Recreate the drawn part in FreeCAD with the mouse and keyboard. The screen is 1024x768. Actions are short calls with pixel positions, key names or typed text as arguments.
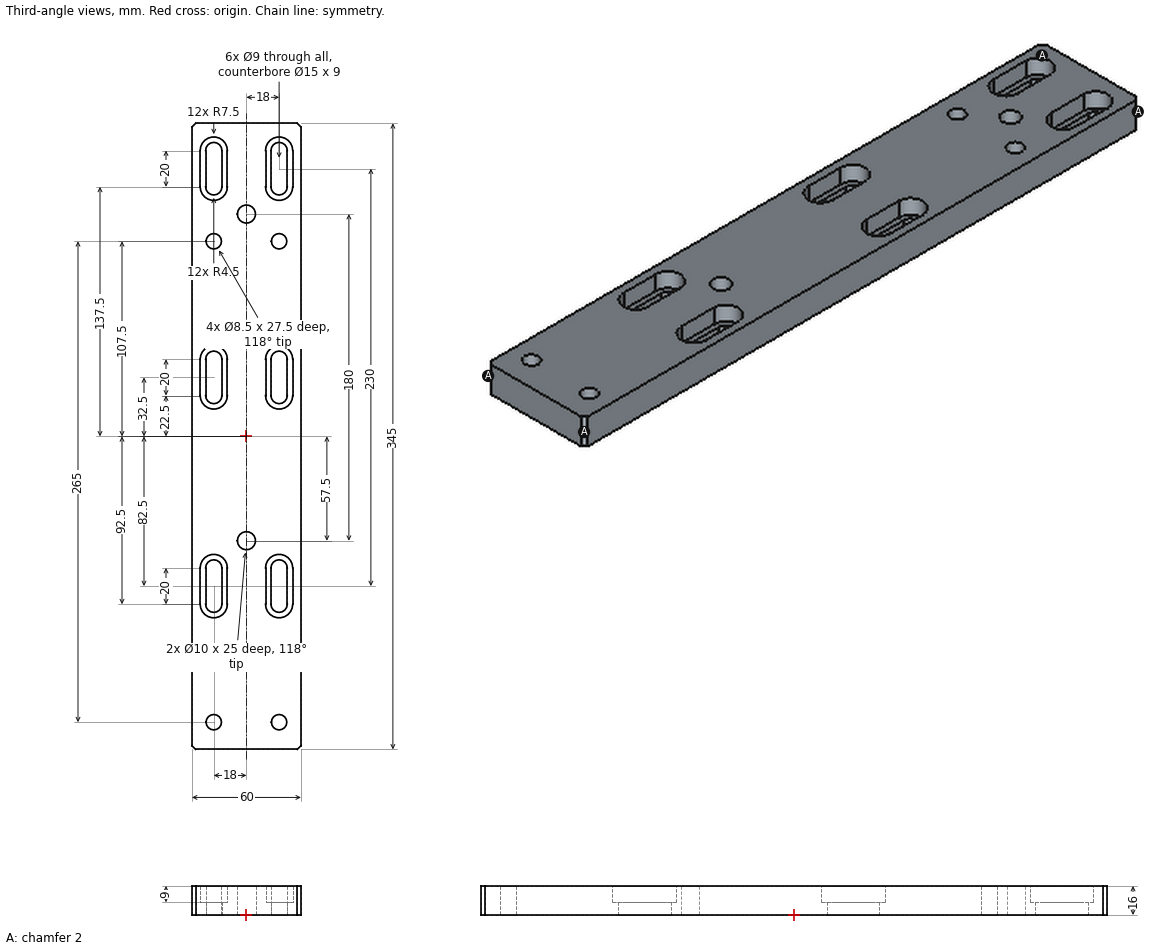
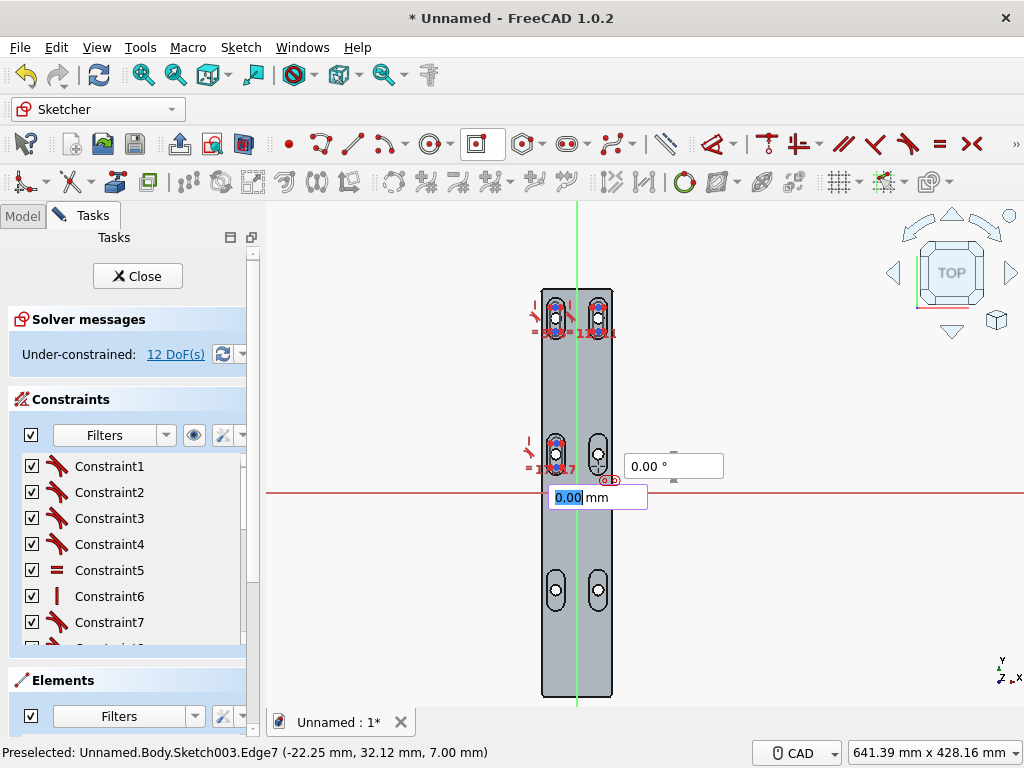
click(598, 443)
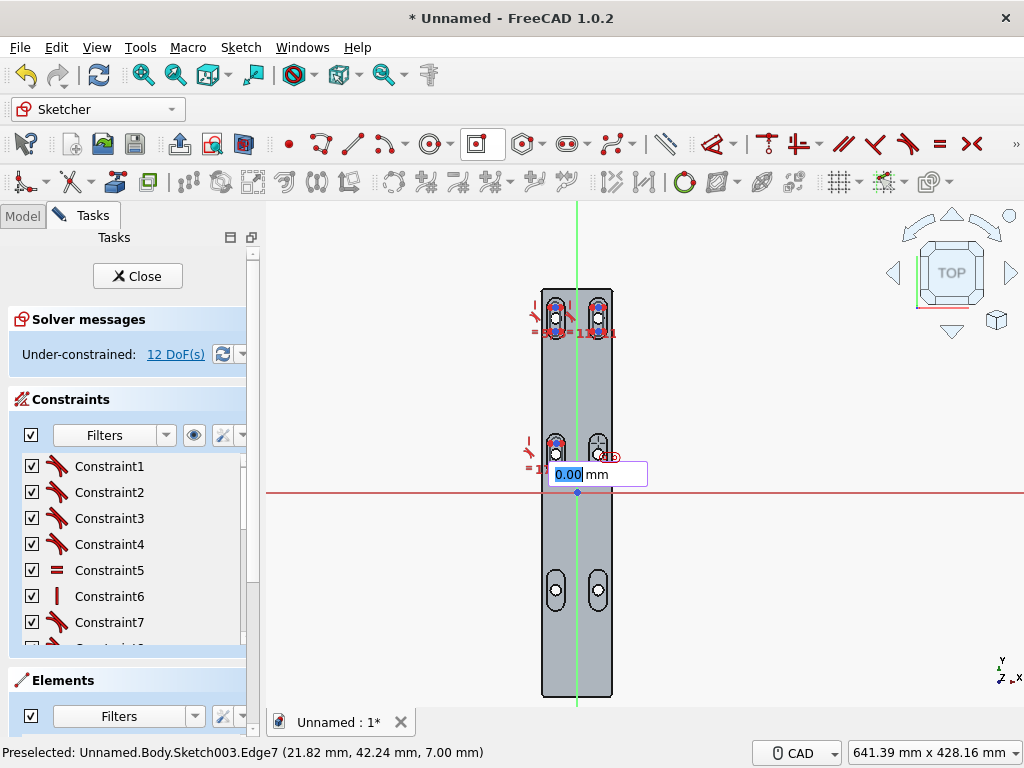
scroll(593, 454, up, 6)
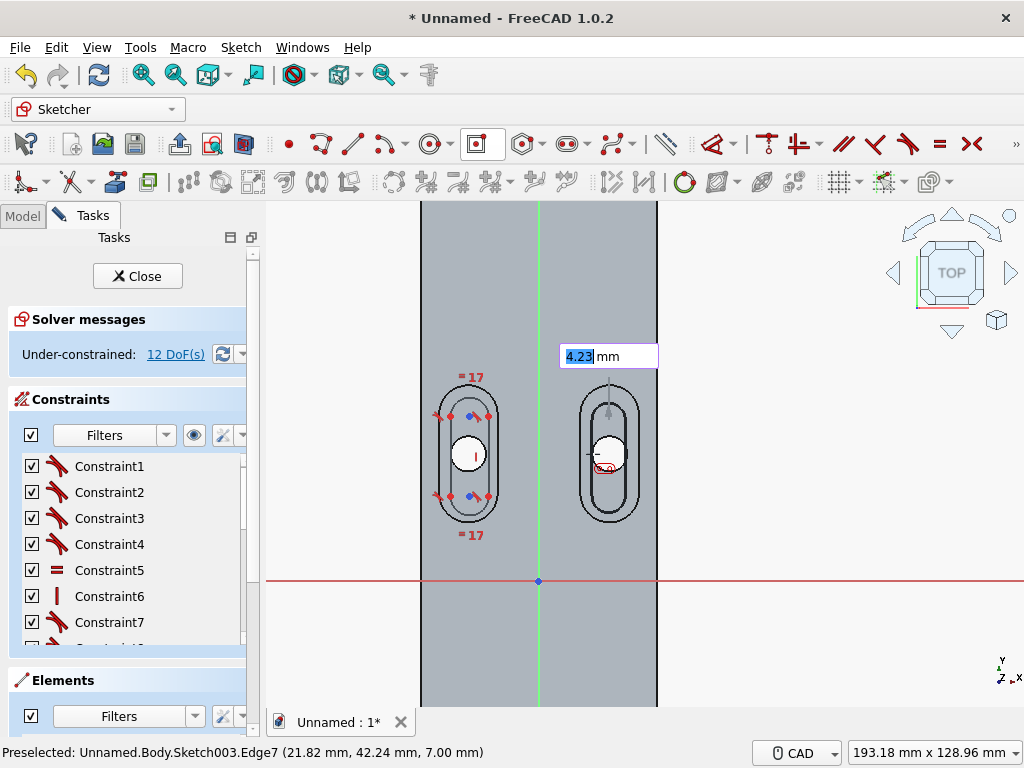
click(592, 454)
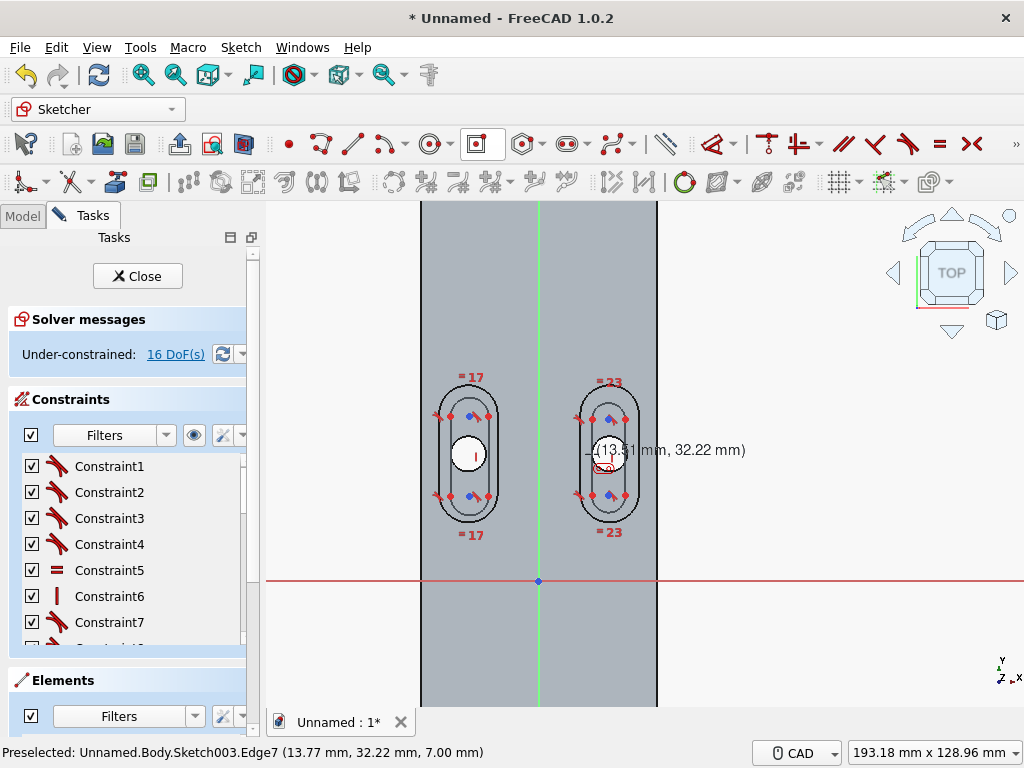
scroll(593, 454, down, 6)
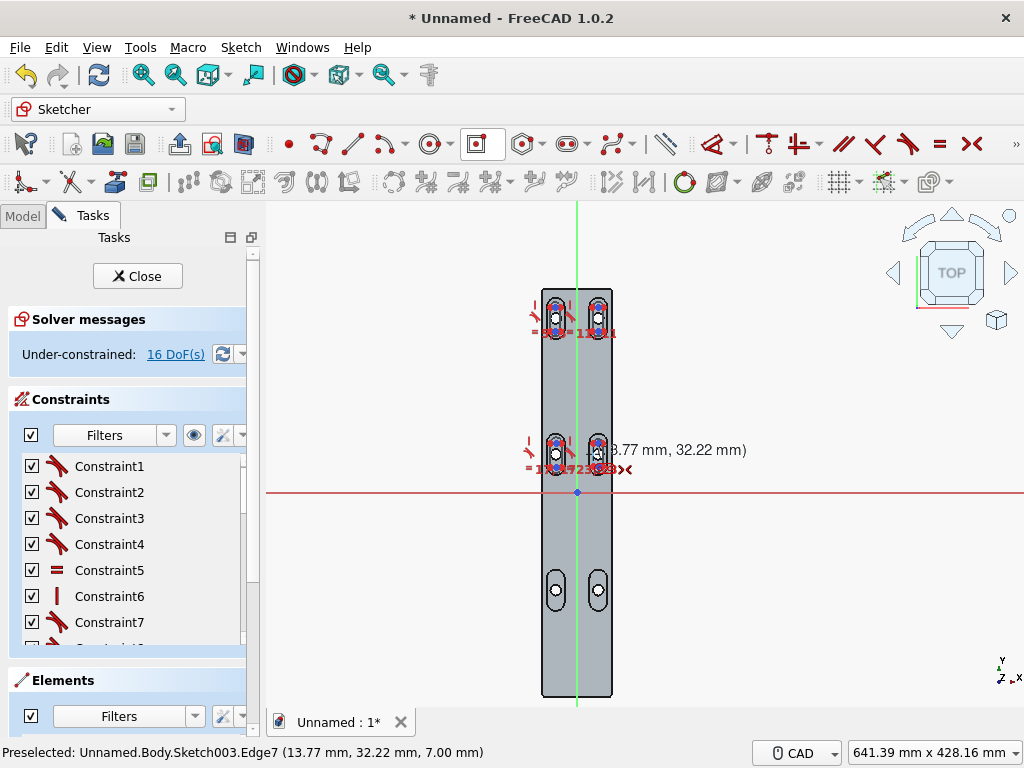
scroll(556, 602, up, 8)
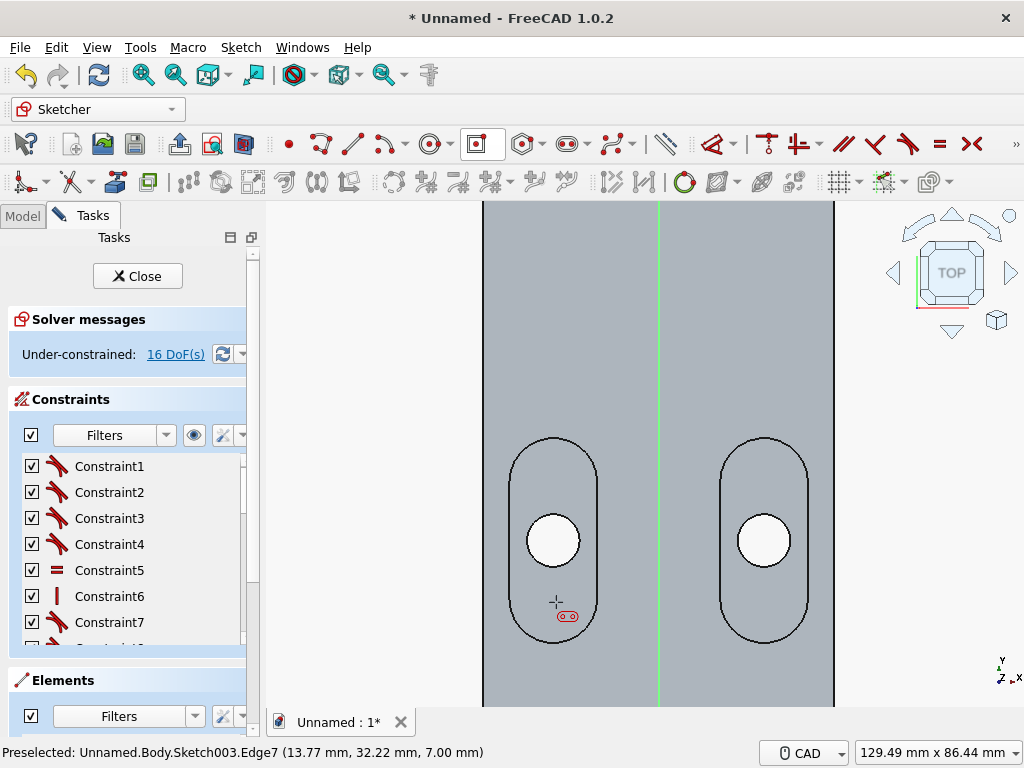
scroll(556, 602, down, 8)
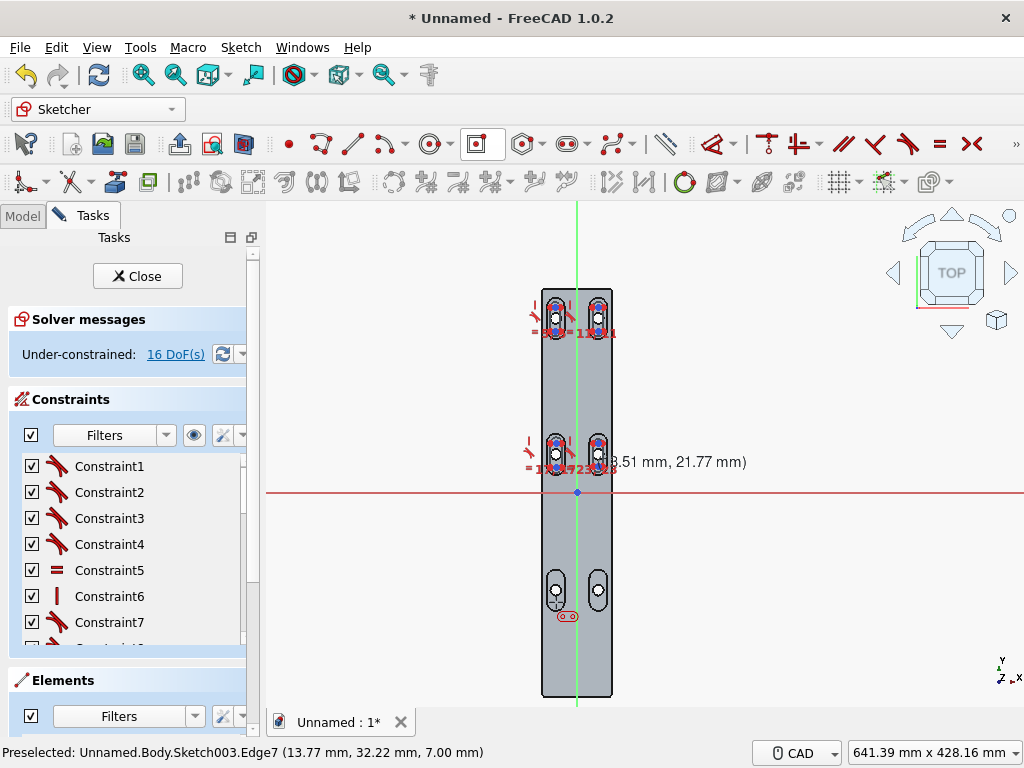
click(556, 602)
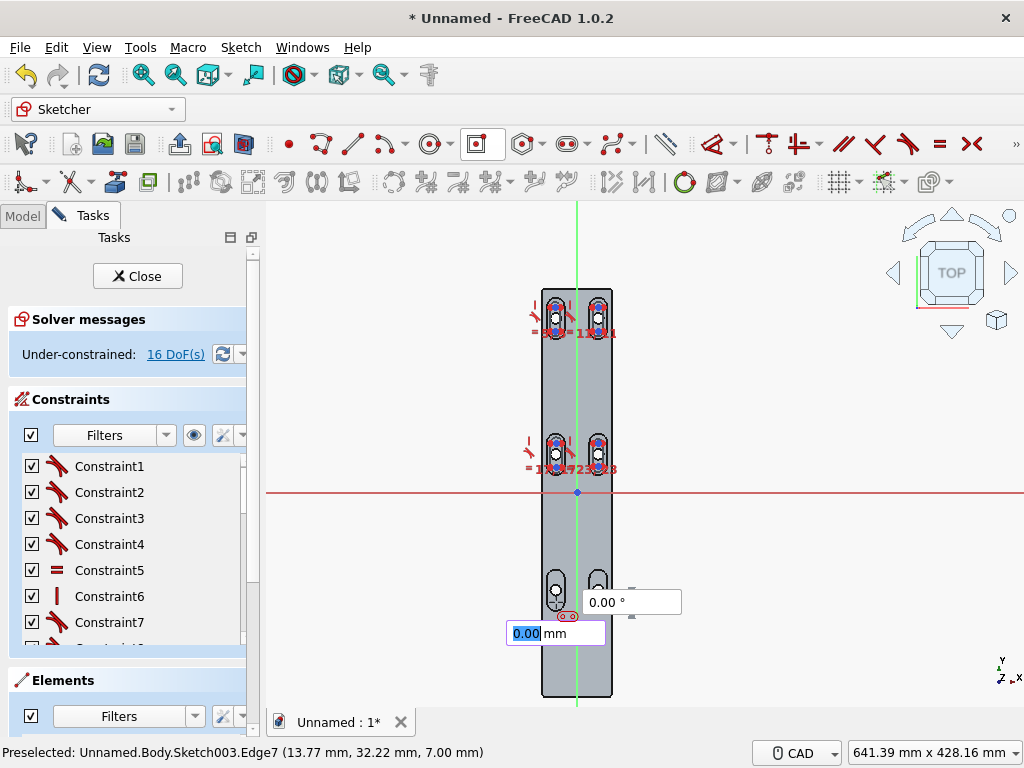
click(556, 578)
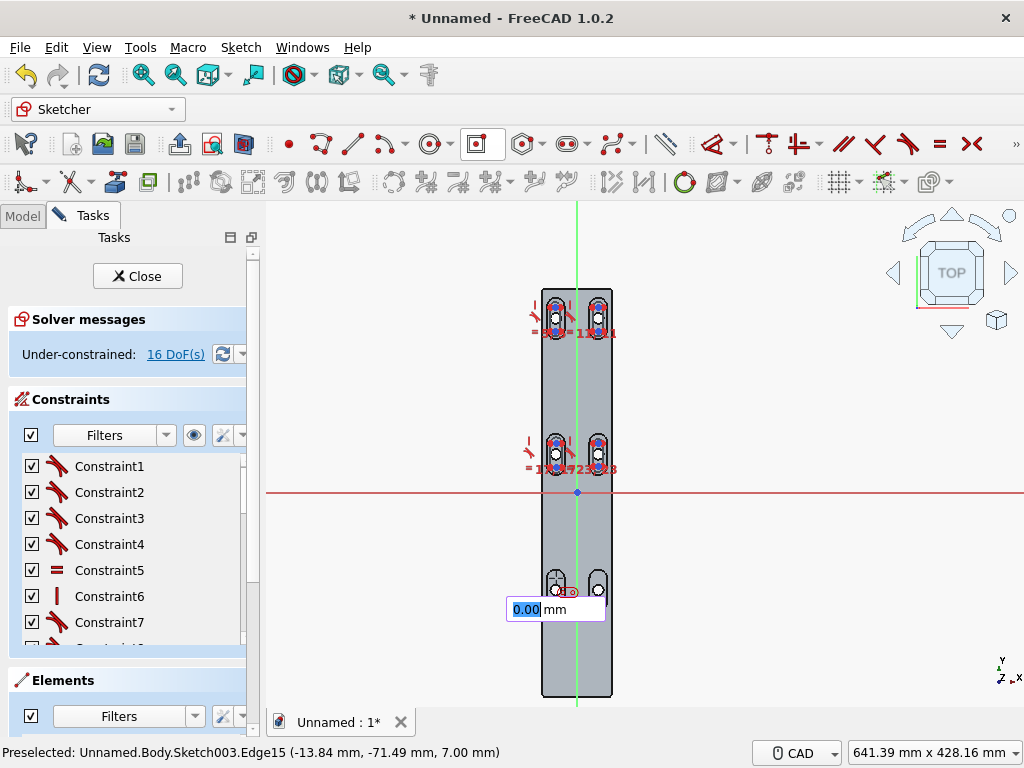
scroll(550, 590, up, 6)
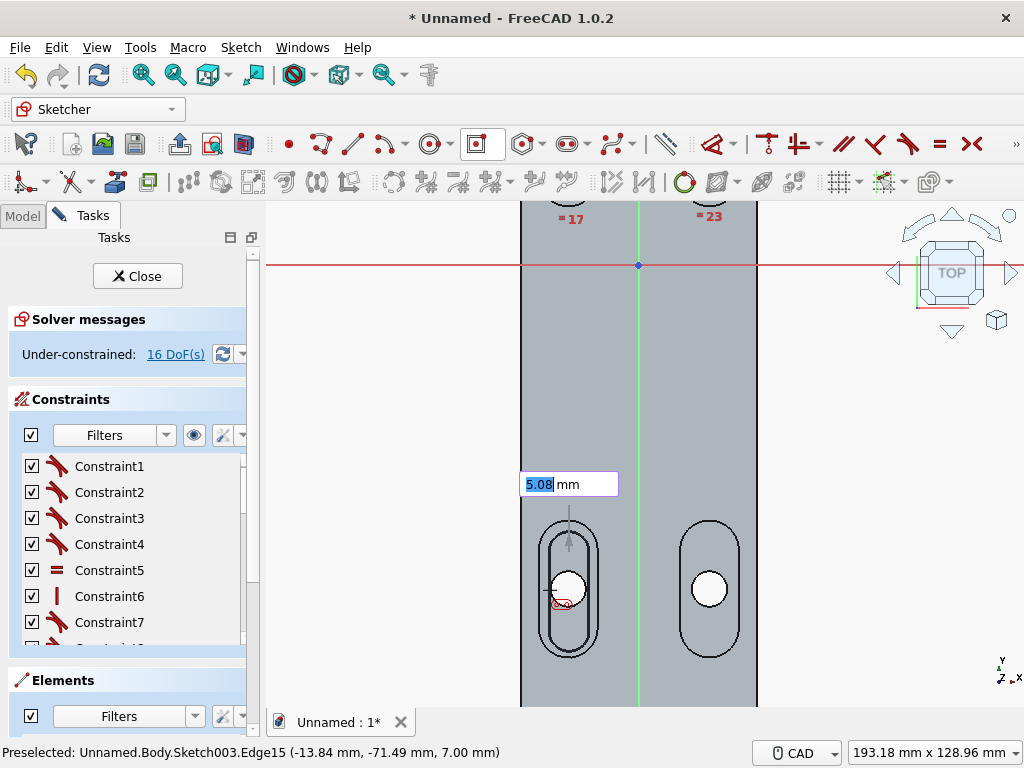
click(551, 589)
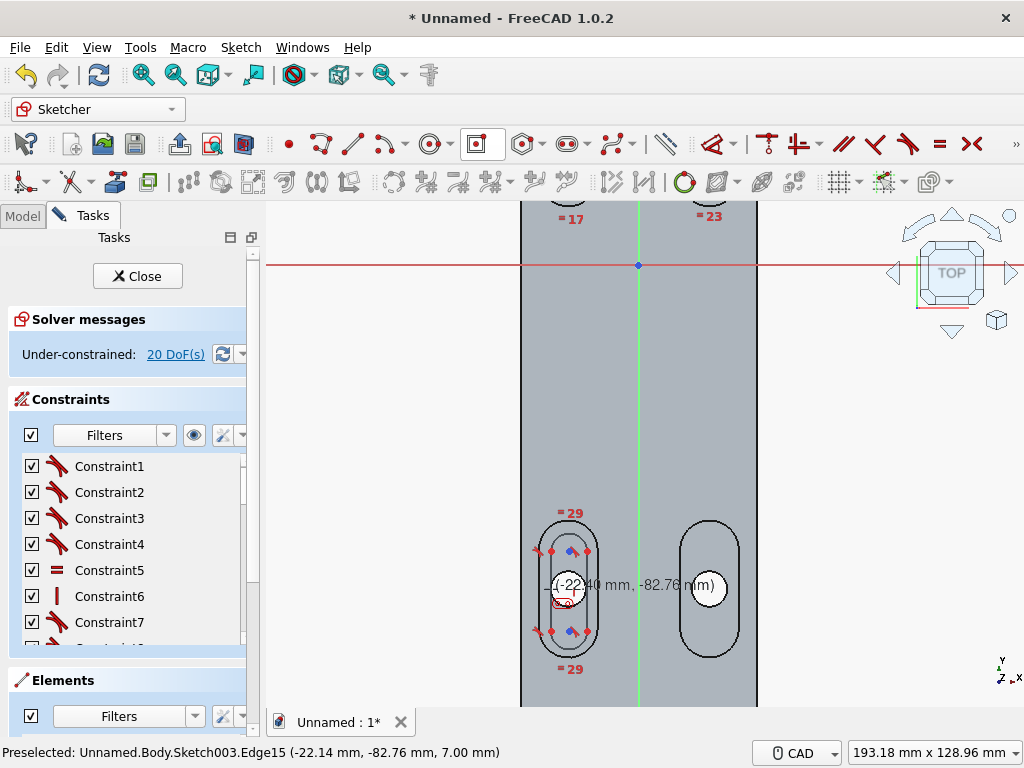
scroll(710, 628, up, 2)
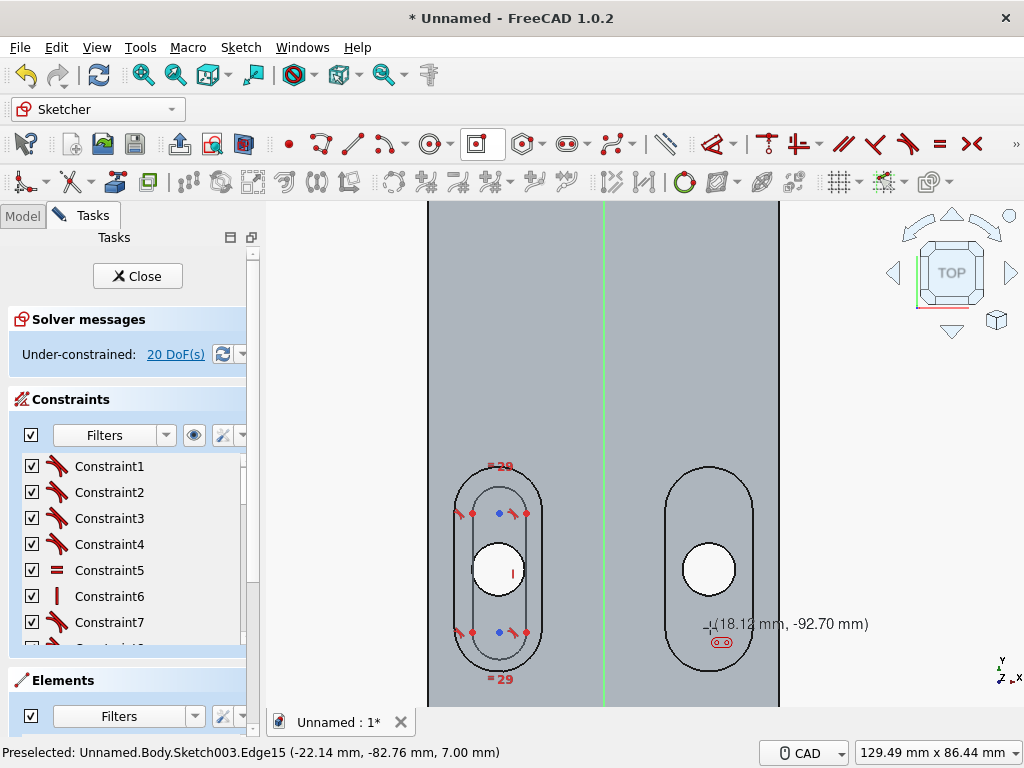
scroll(570, 595, down, 8)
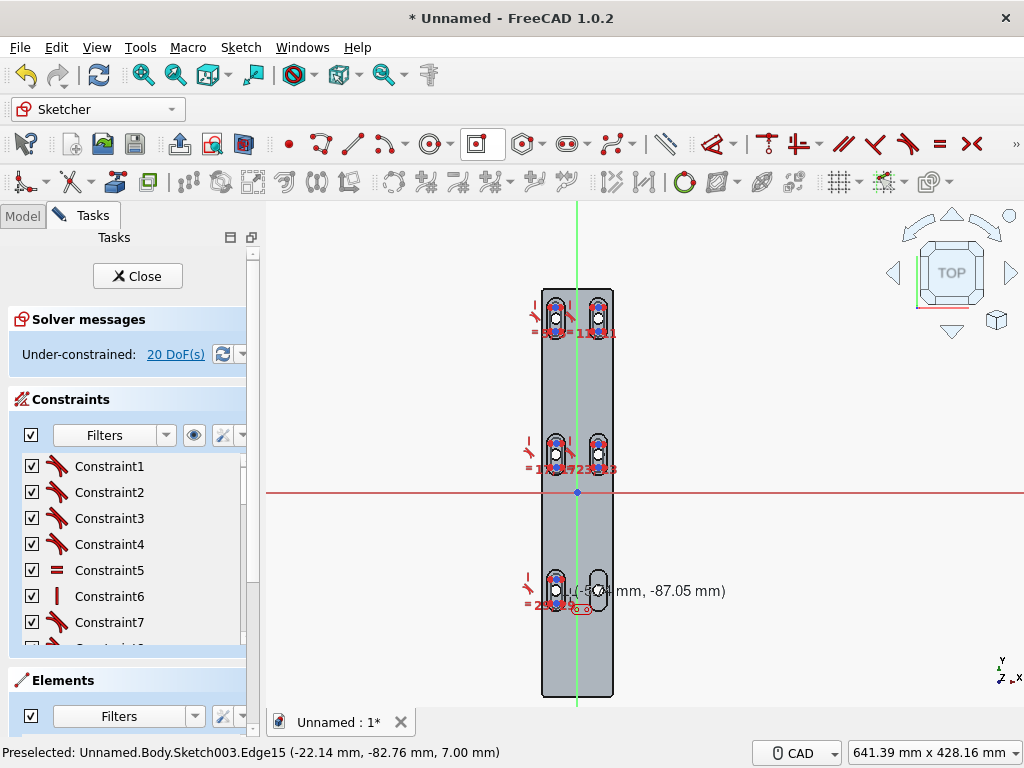
click(598, 602)